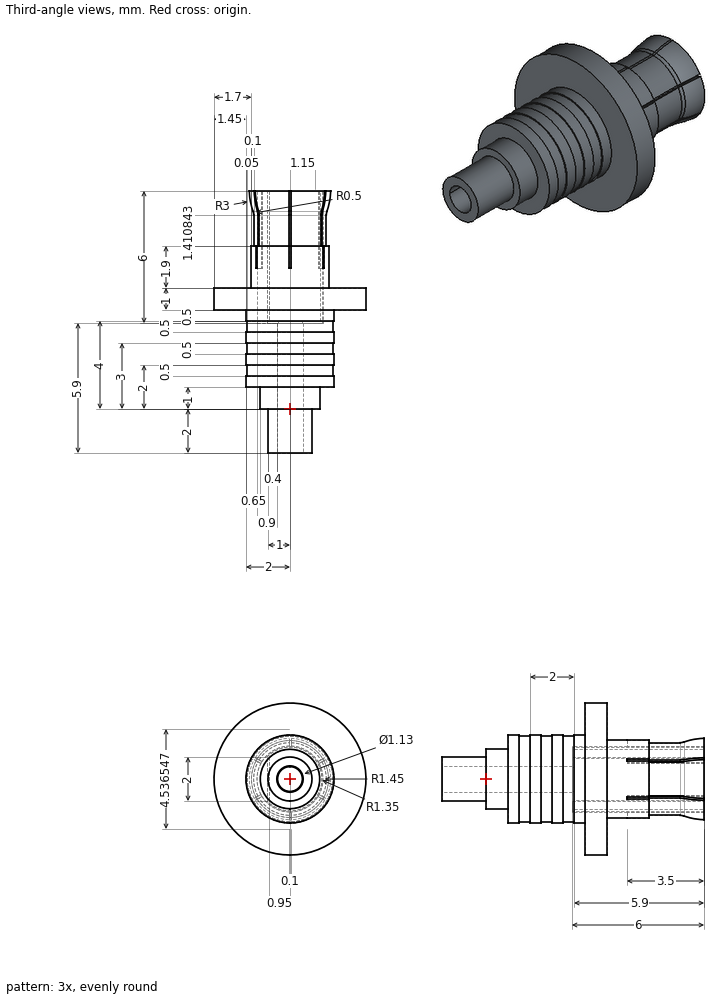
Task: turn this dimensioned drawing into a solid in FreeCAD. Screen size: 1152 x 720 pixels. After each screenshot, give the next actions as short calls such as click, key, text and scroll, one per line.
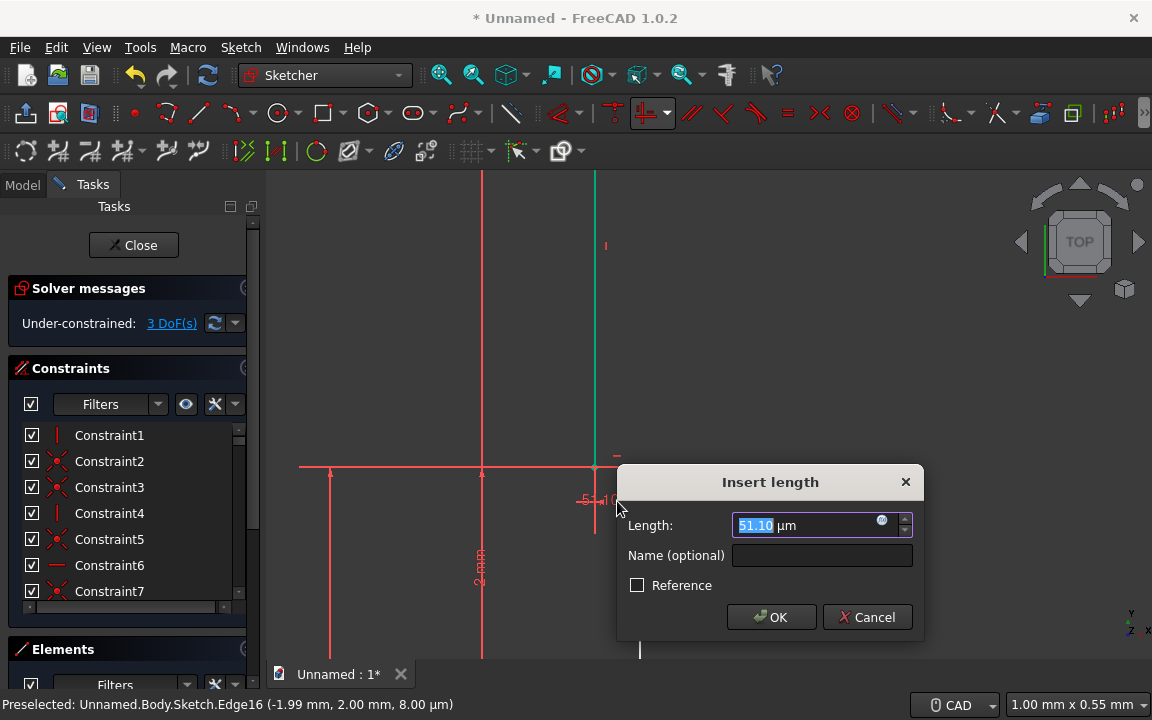
key(ctrl+a)
text(0.05 mm)
key(Return)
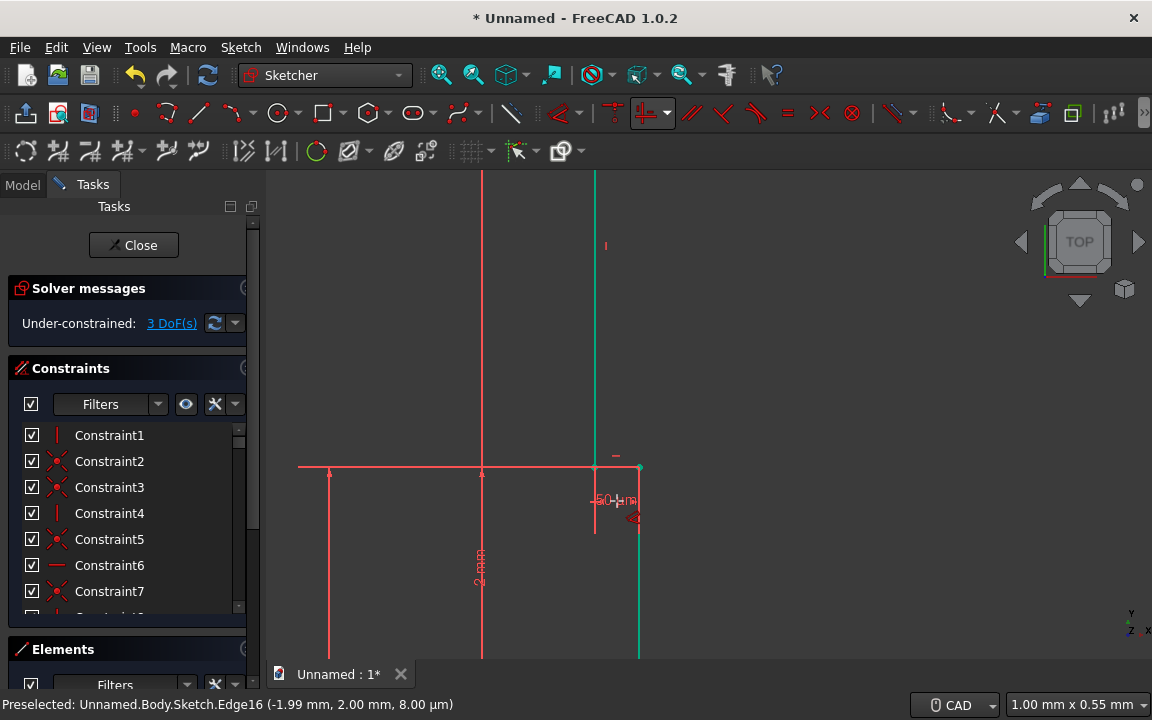
scroll(634, 472, down, 17)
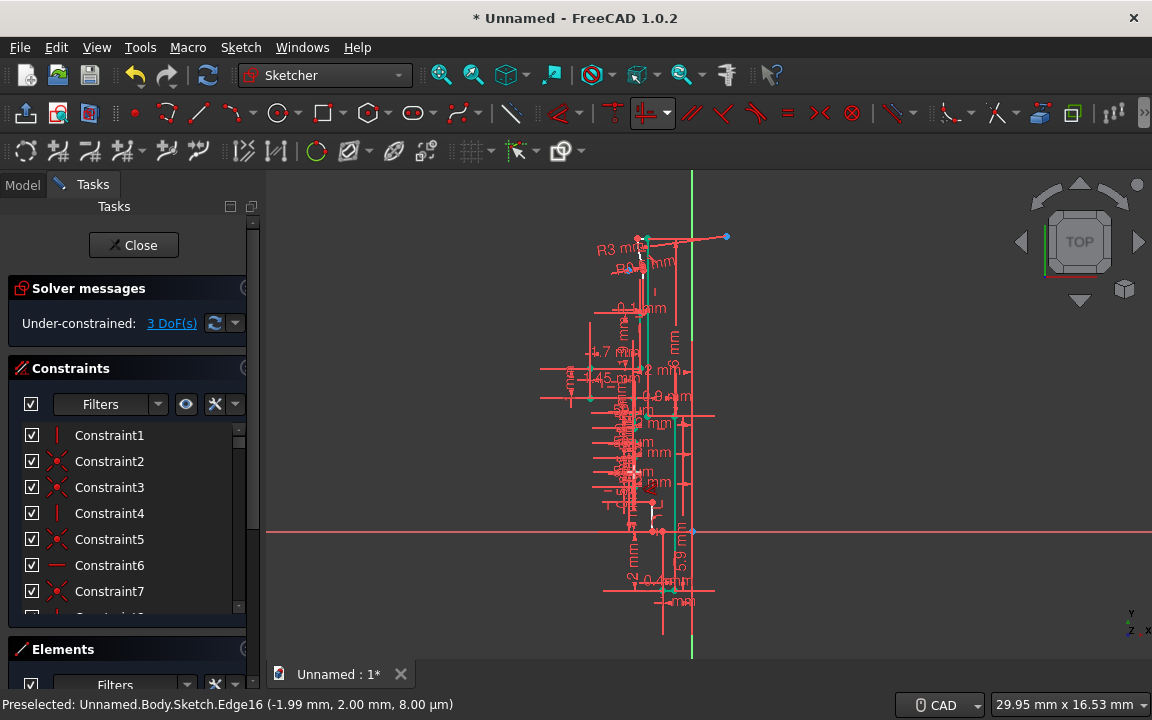
scroll(639, 502, up, 5)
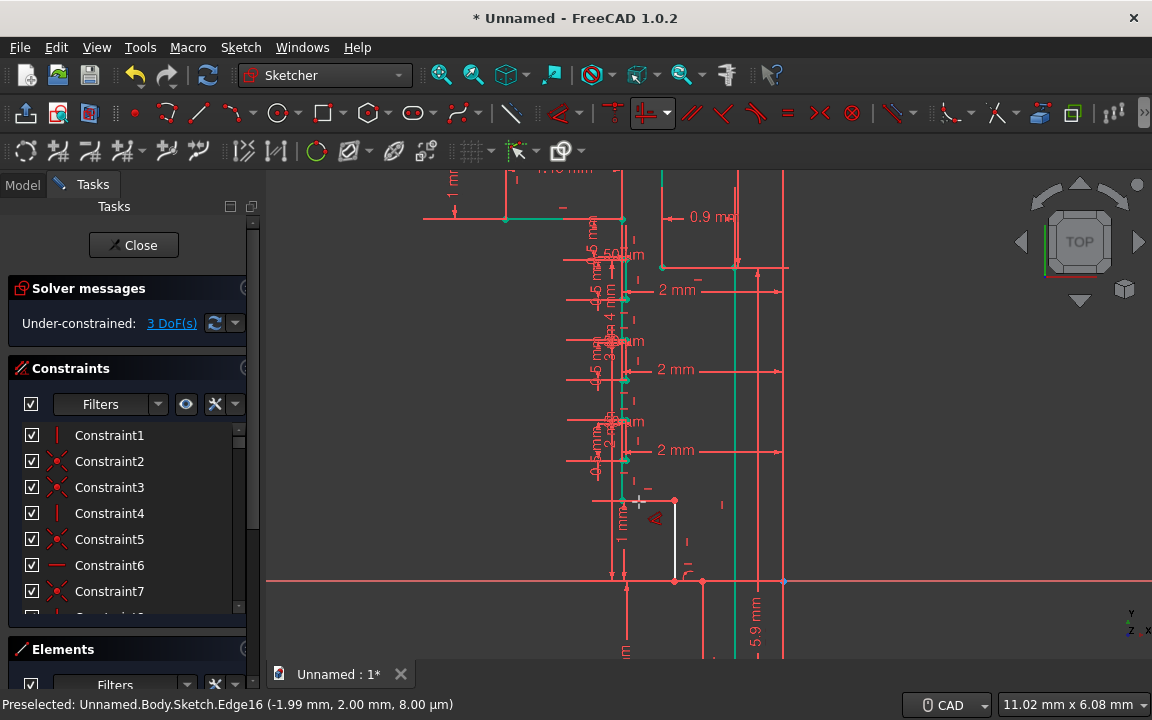
click(638, 501)
click(649, 559)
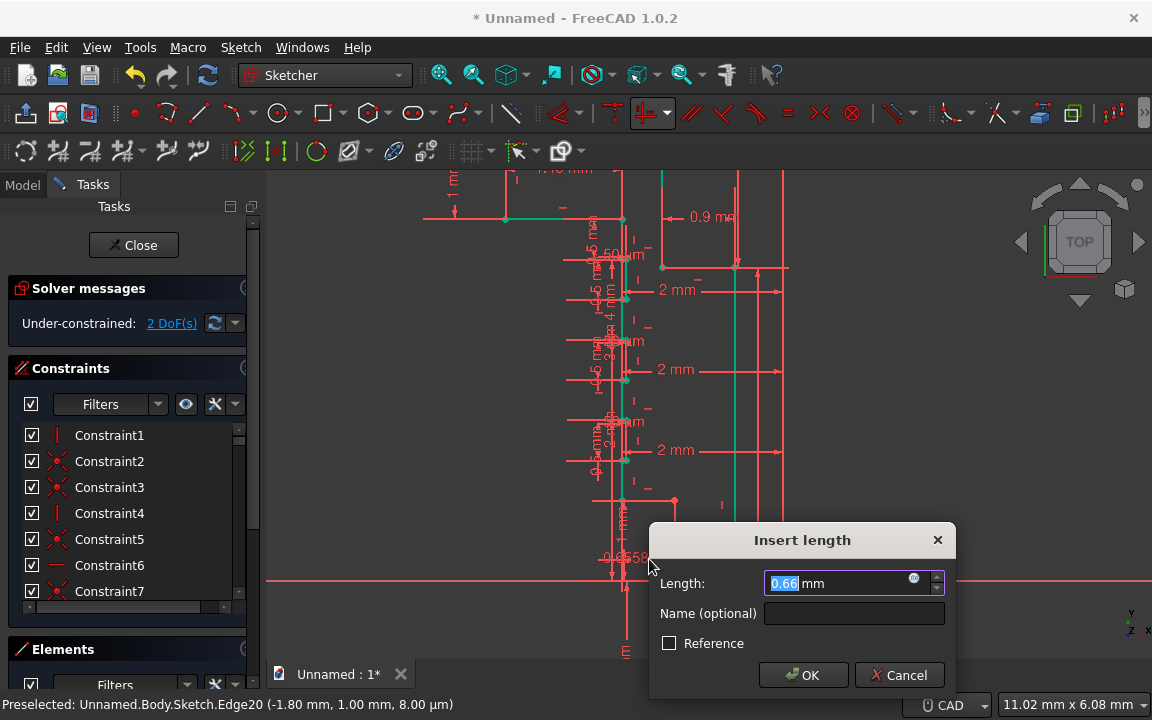
text(0.65)
key(Return)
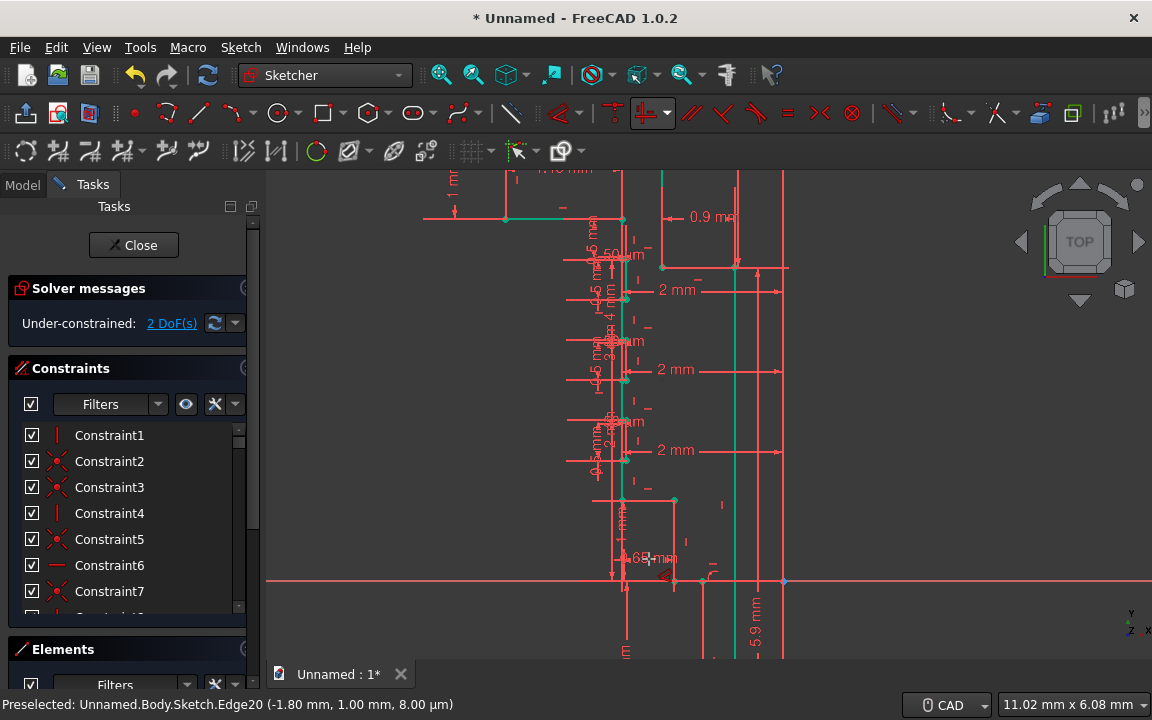
scroll(639, 480, down, 6)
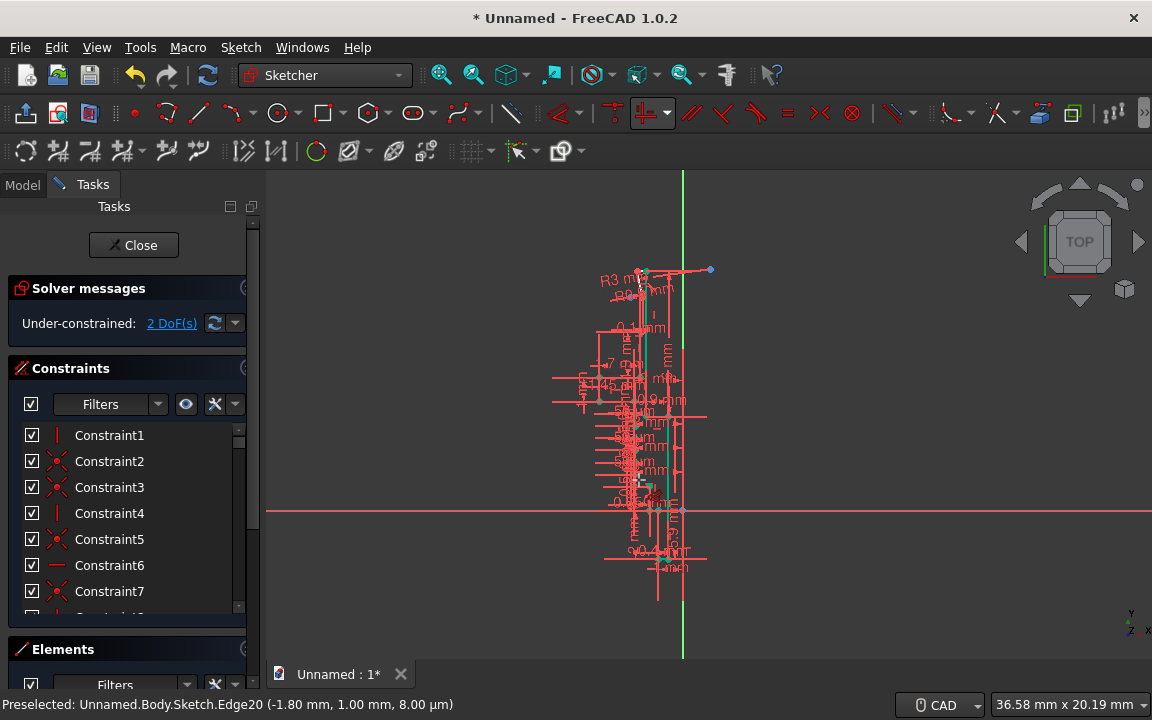
scroll(711, 269, up, 2)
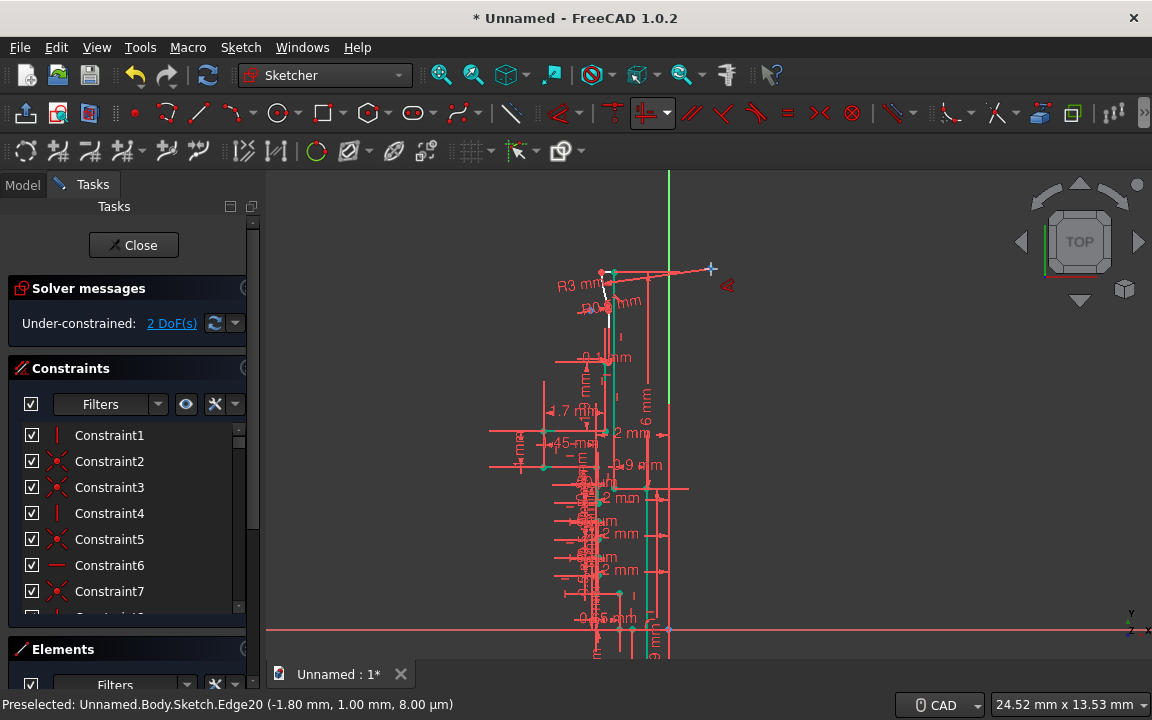
click(710, 269)
click(689, 235)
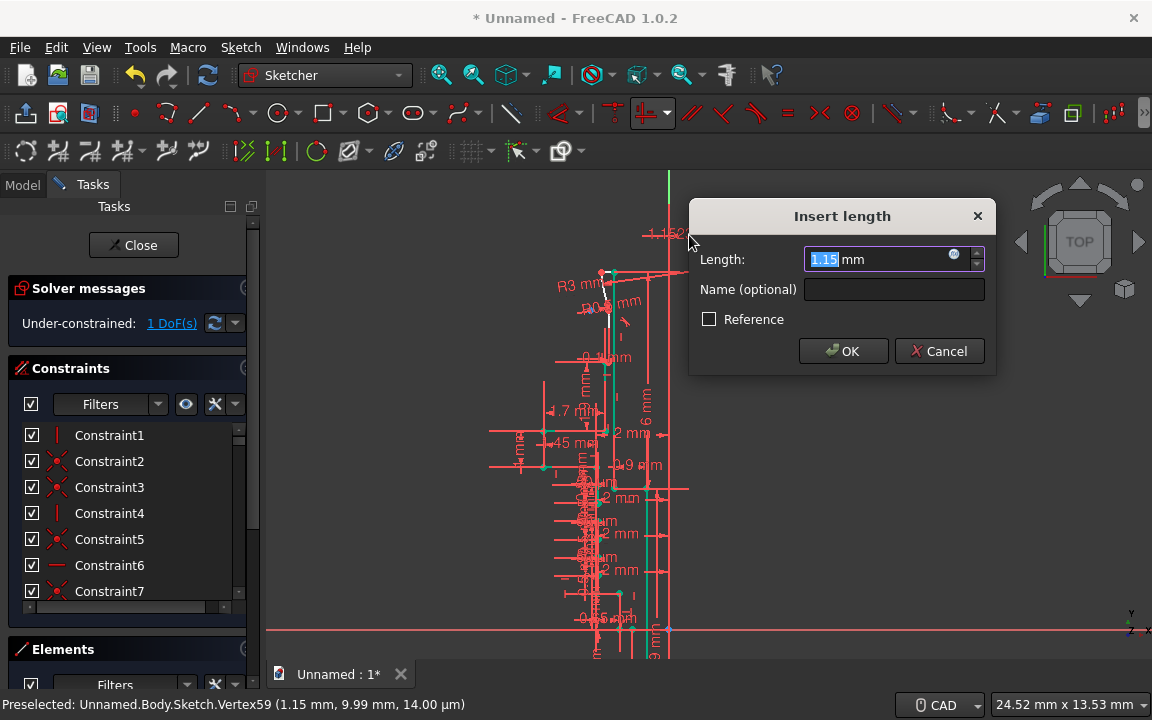
text(1.15)
key(Return)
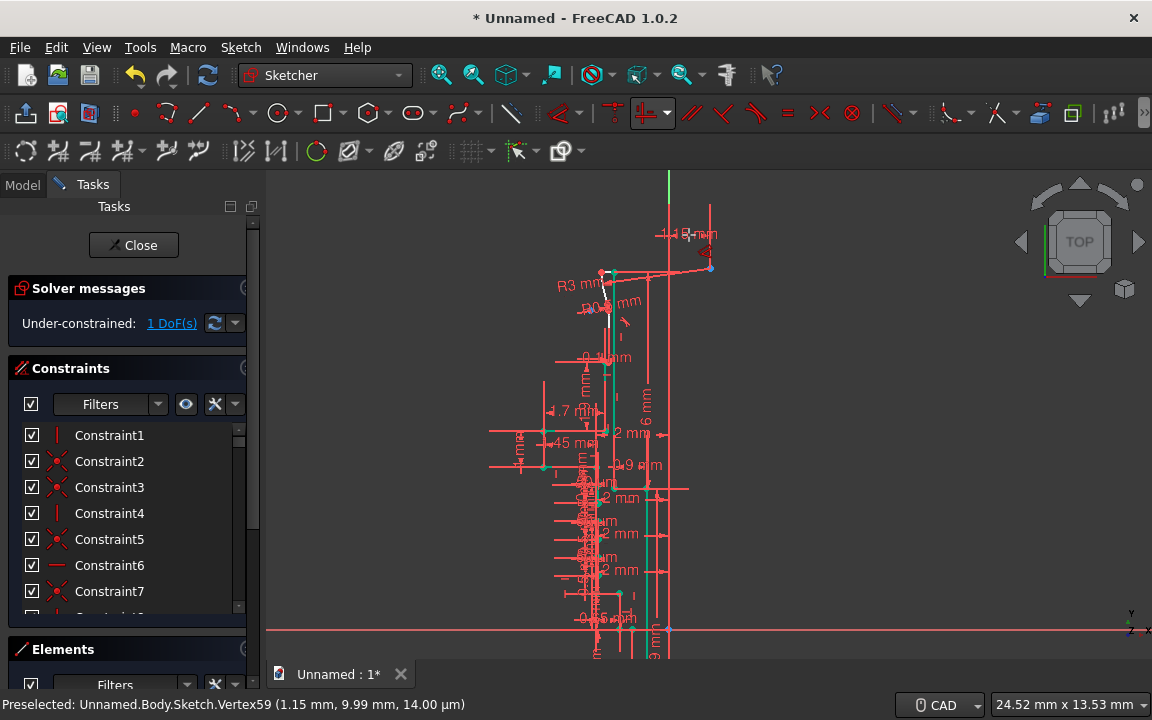
scroll(609, 326, up, 5)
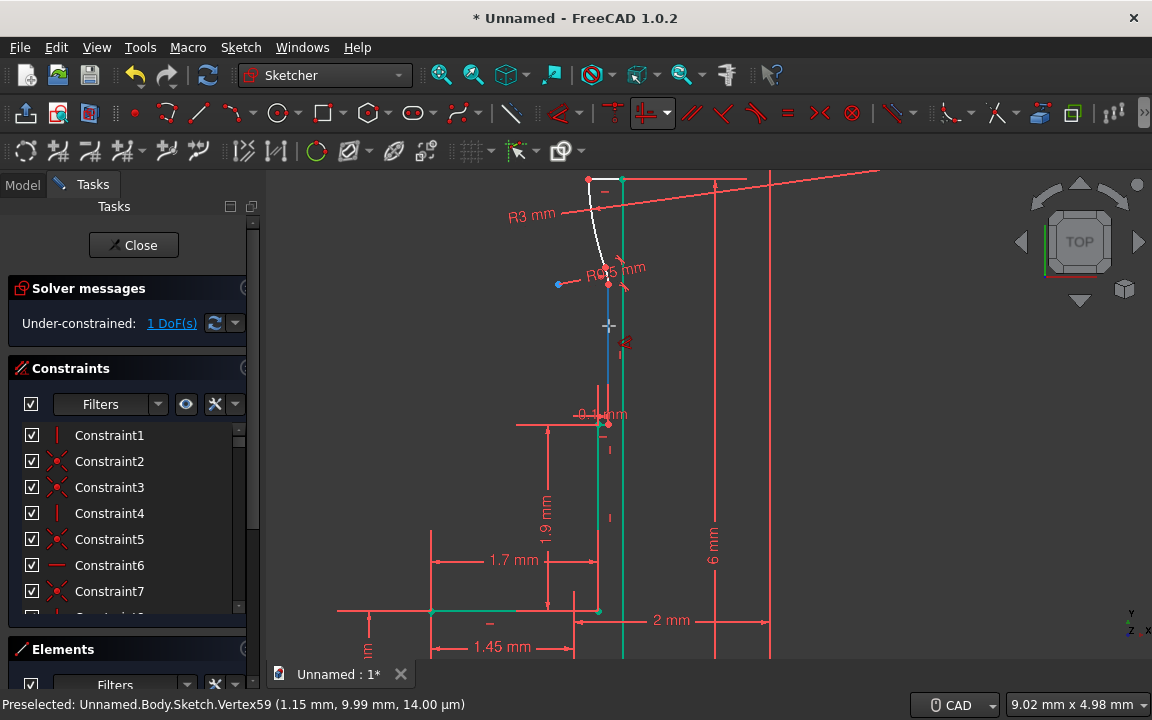
click(608, 326)
click(642, 354)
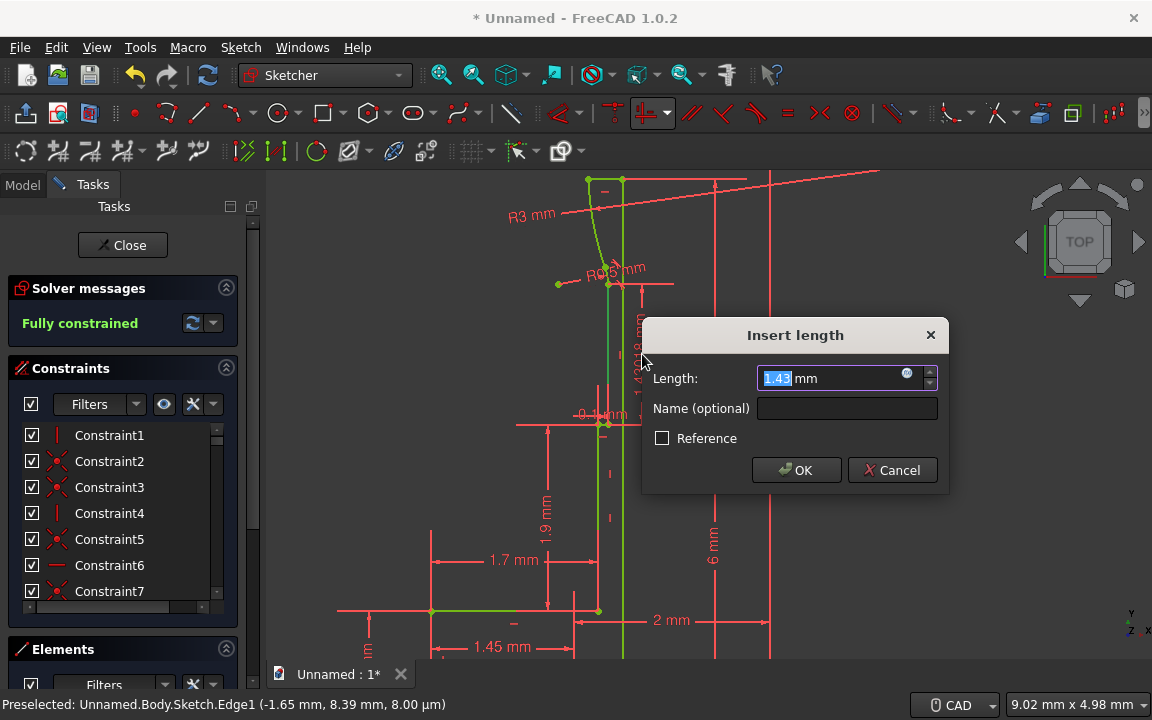
text(1.410843)
key(Return)
key(Escape)